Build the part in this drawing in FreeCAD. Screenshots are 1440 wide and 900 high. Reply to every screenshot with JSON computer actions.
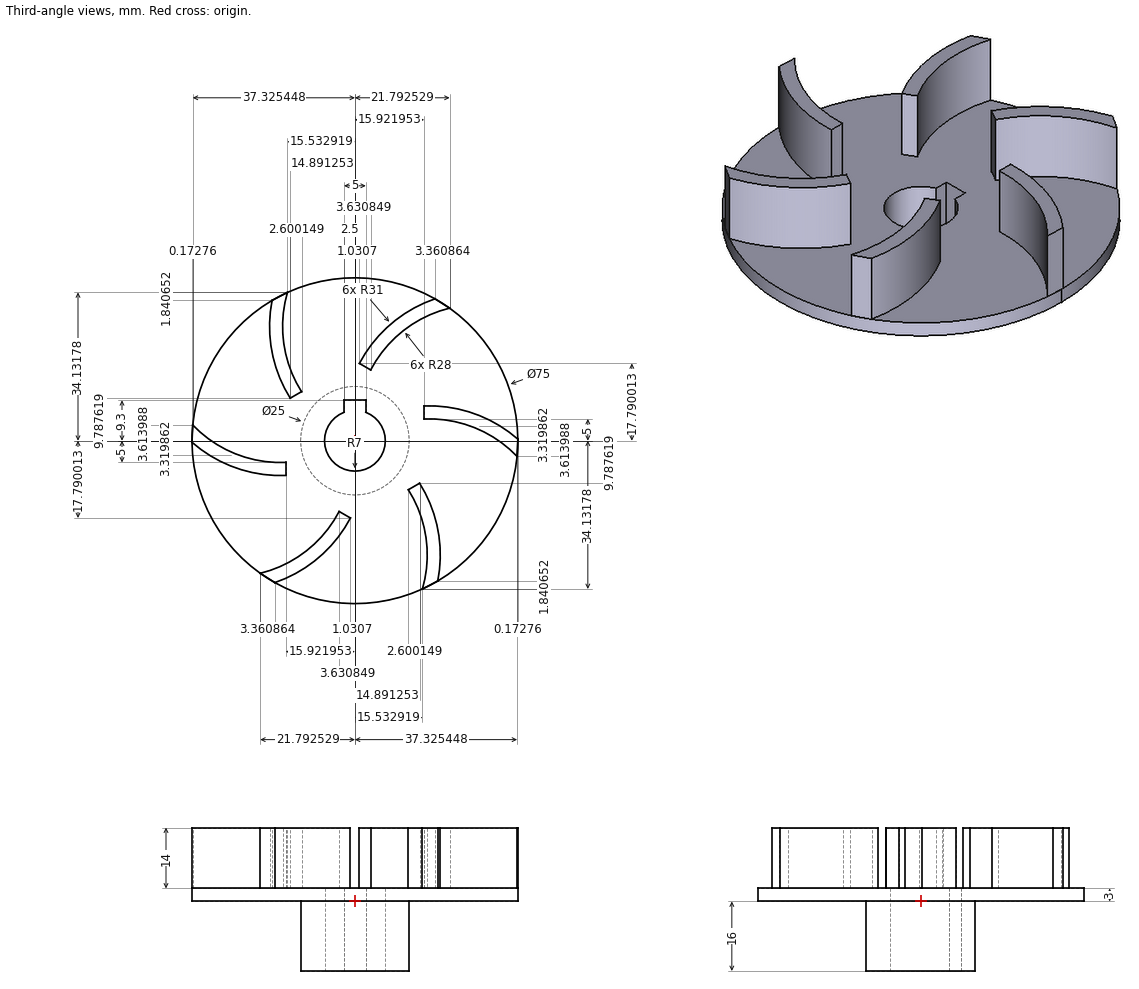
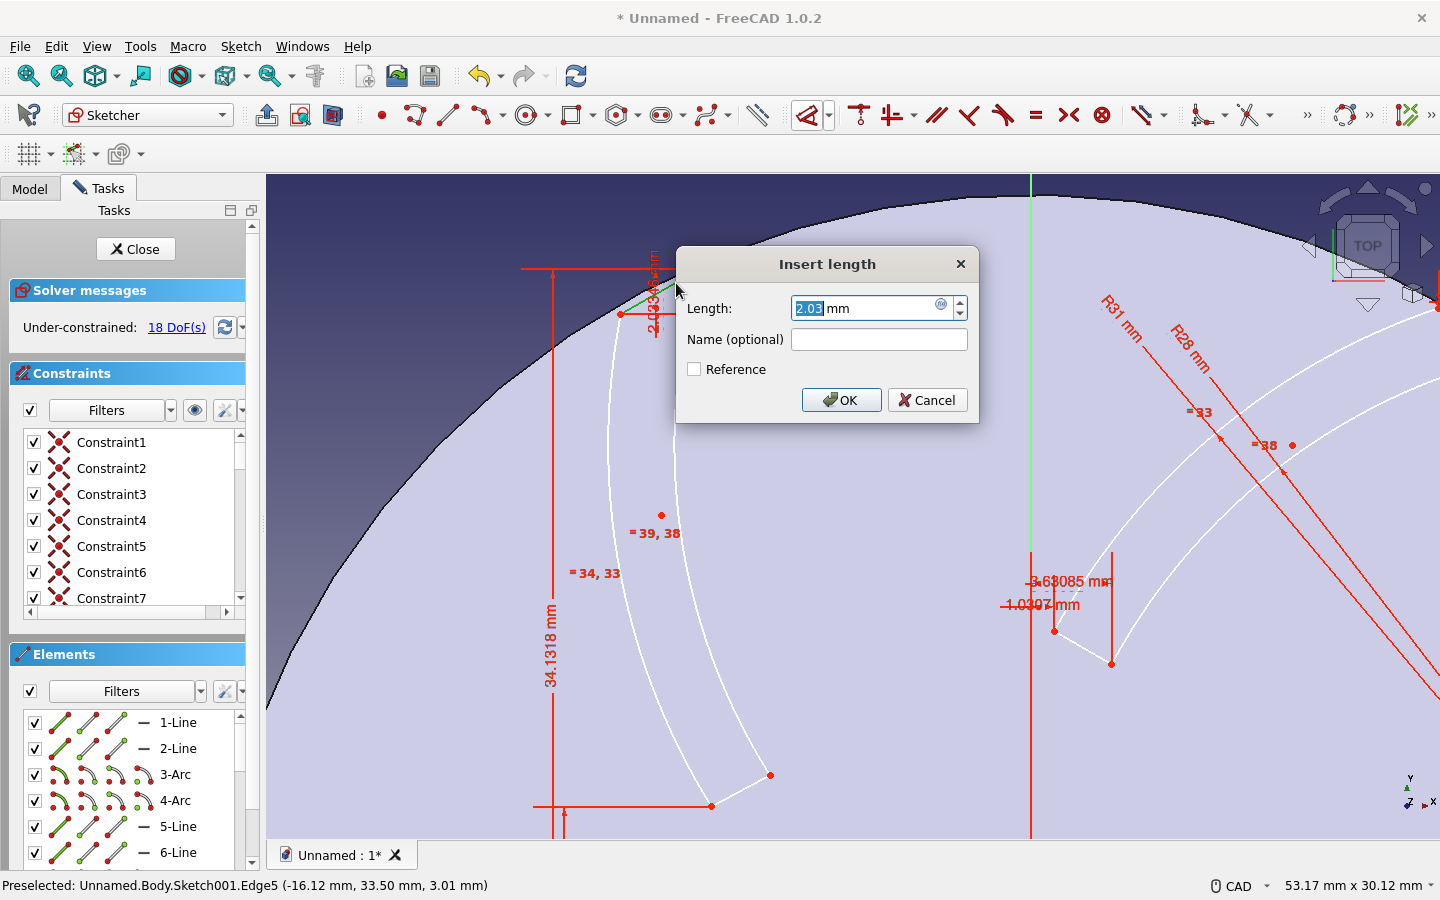
{"action": "type", "text": "1.840652"}
{"action": "key", "text": "Return"}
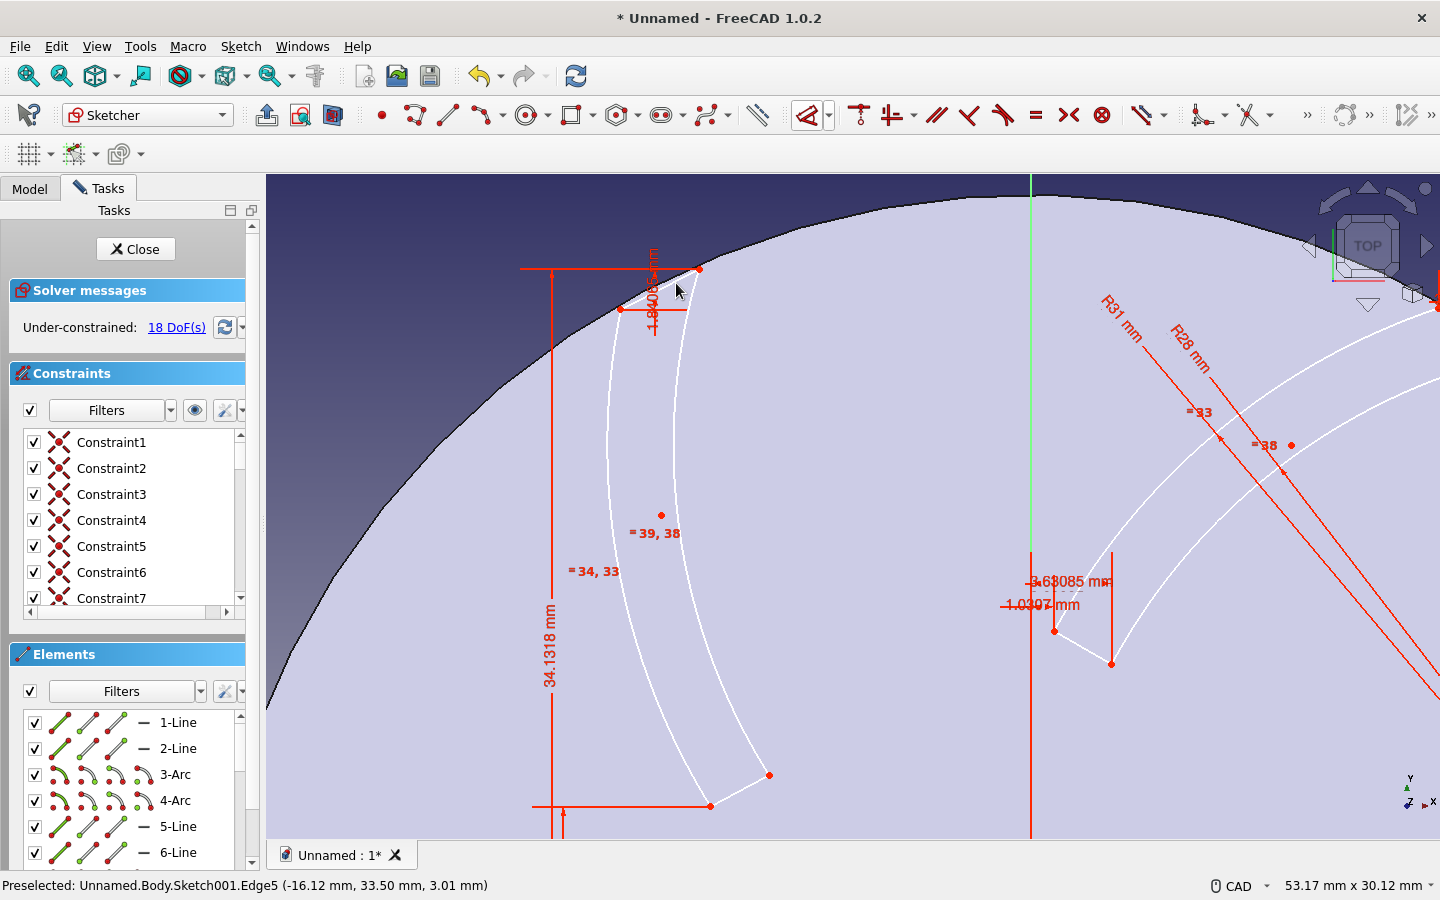
{"action": "left_click", "coordinate": [728, 797]}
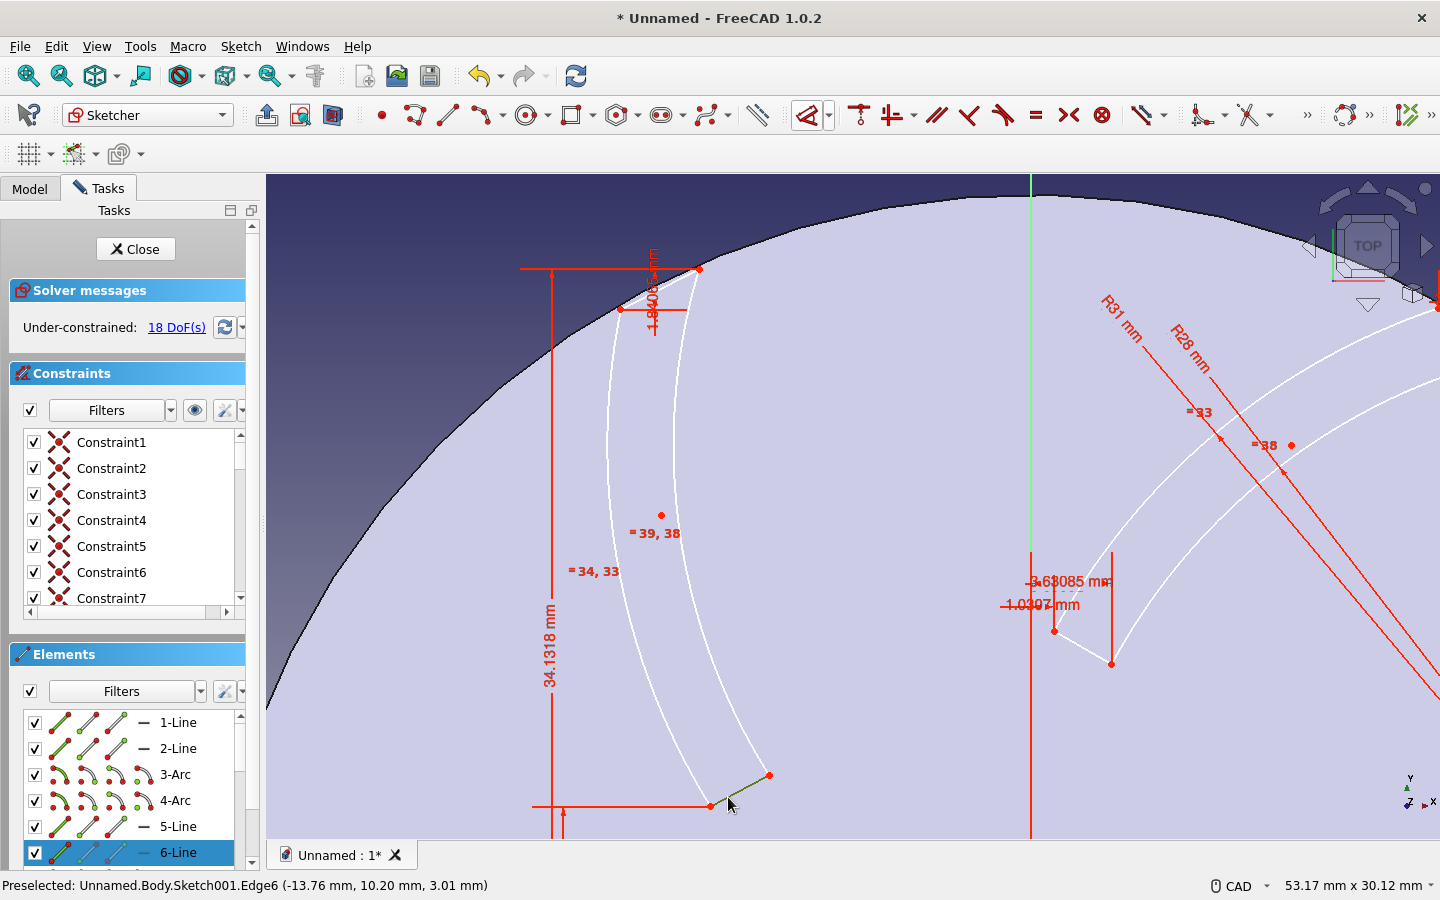
{"action": "key", "text": "l"}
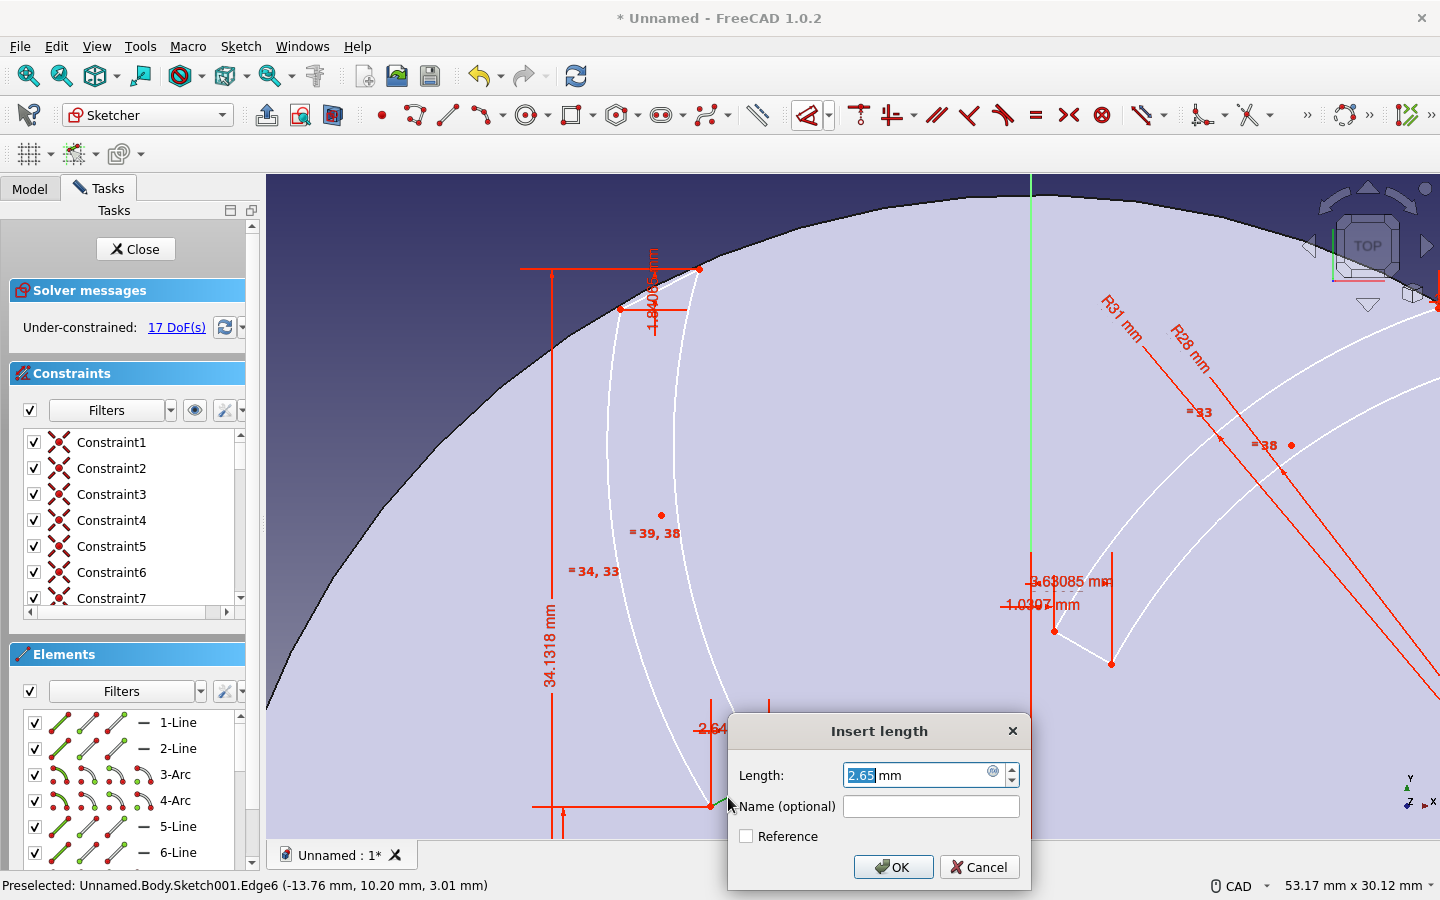
{"action": "type", "text": "2.600149"}
{"action": "key", "text": "Return"}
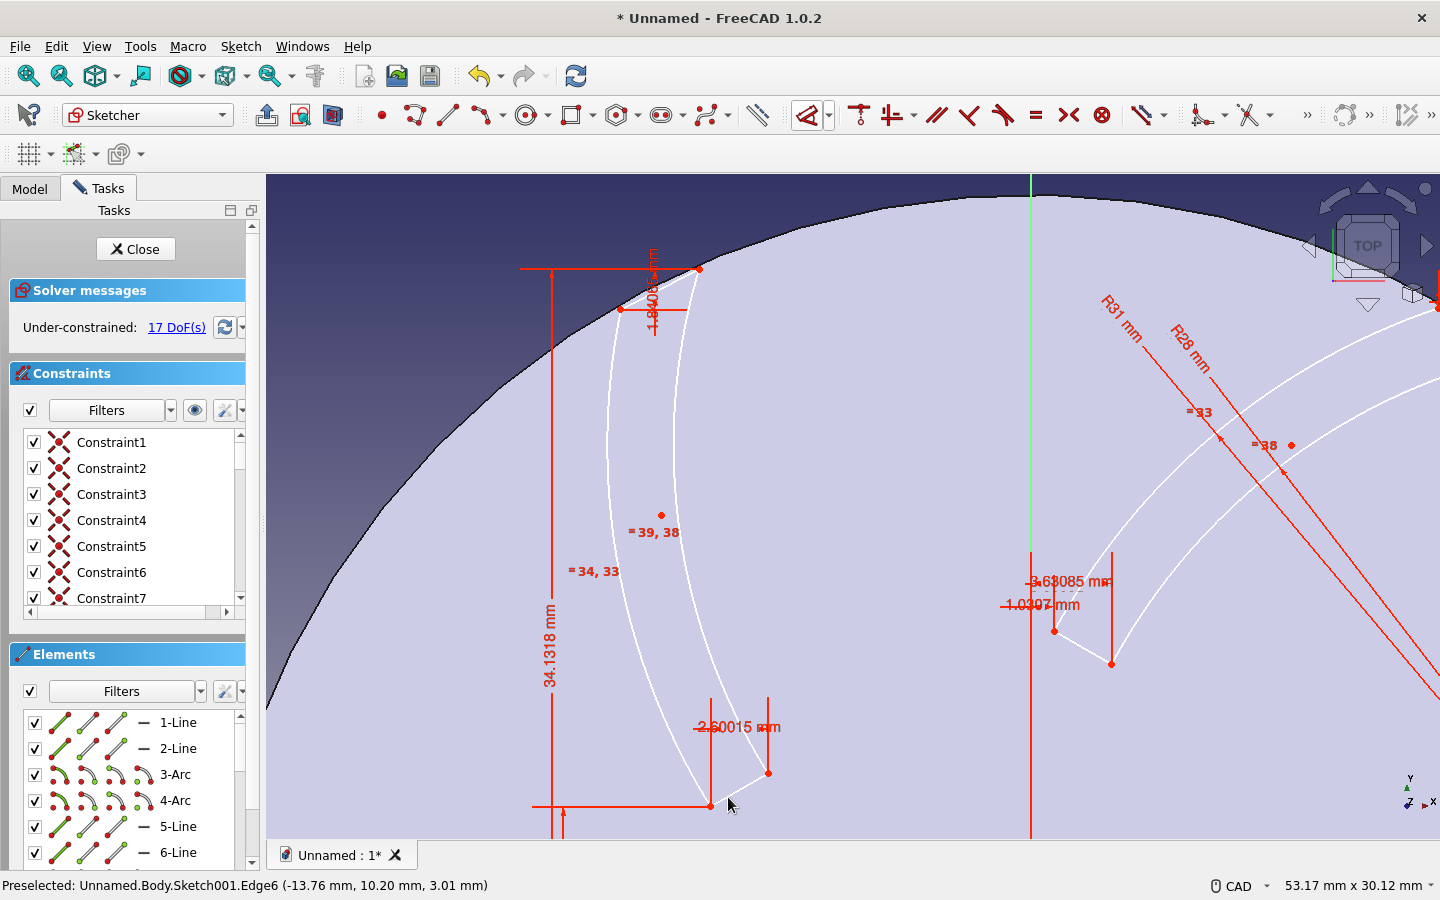
{"action": "scroll", "coordinate": [678, 284], "scroll_direction": "down", "scroll_amount": 6}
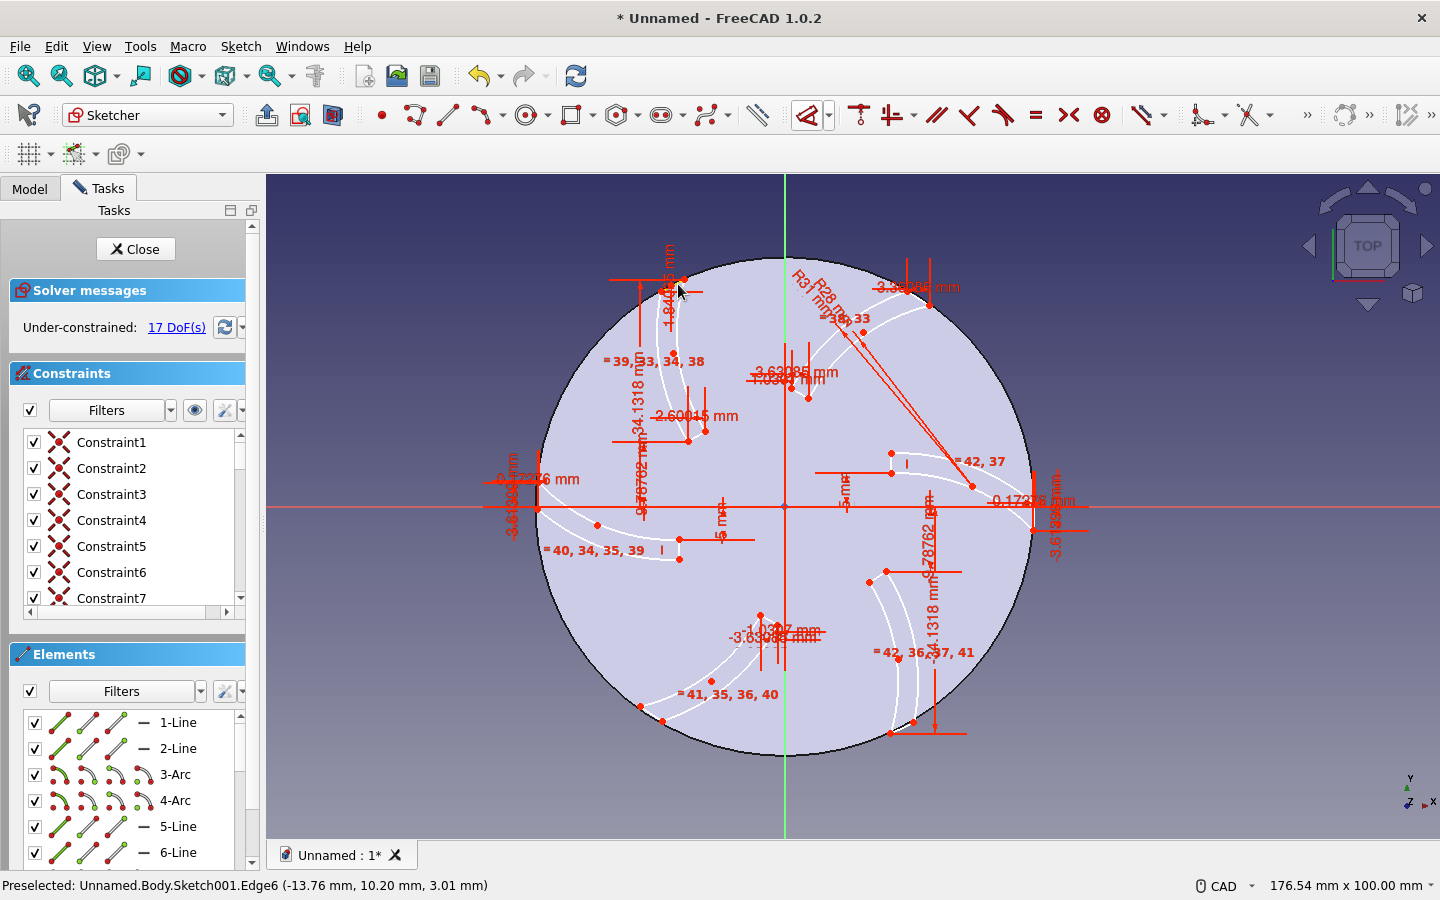
{"action": "scroll", "coordinate": [647, 711], "scroll_direction": "up", "scroll_amount": 5}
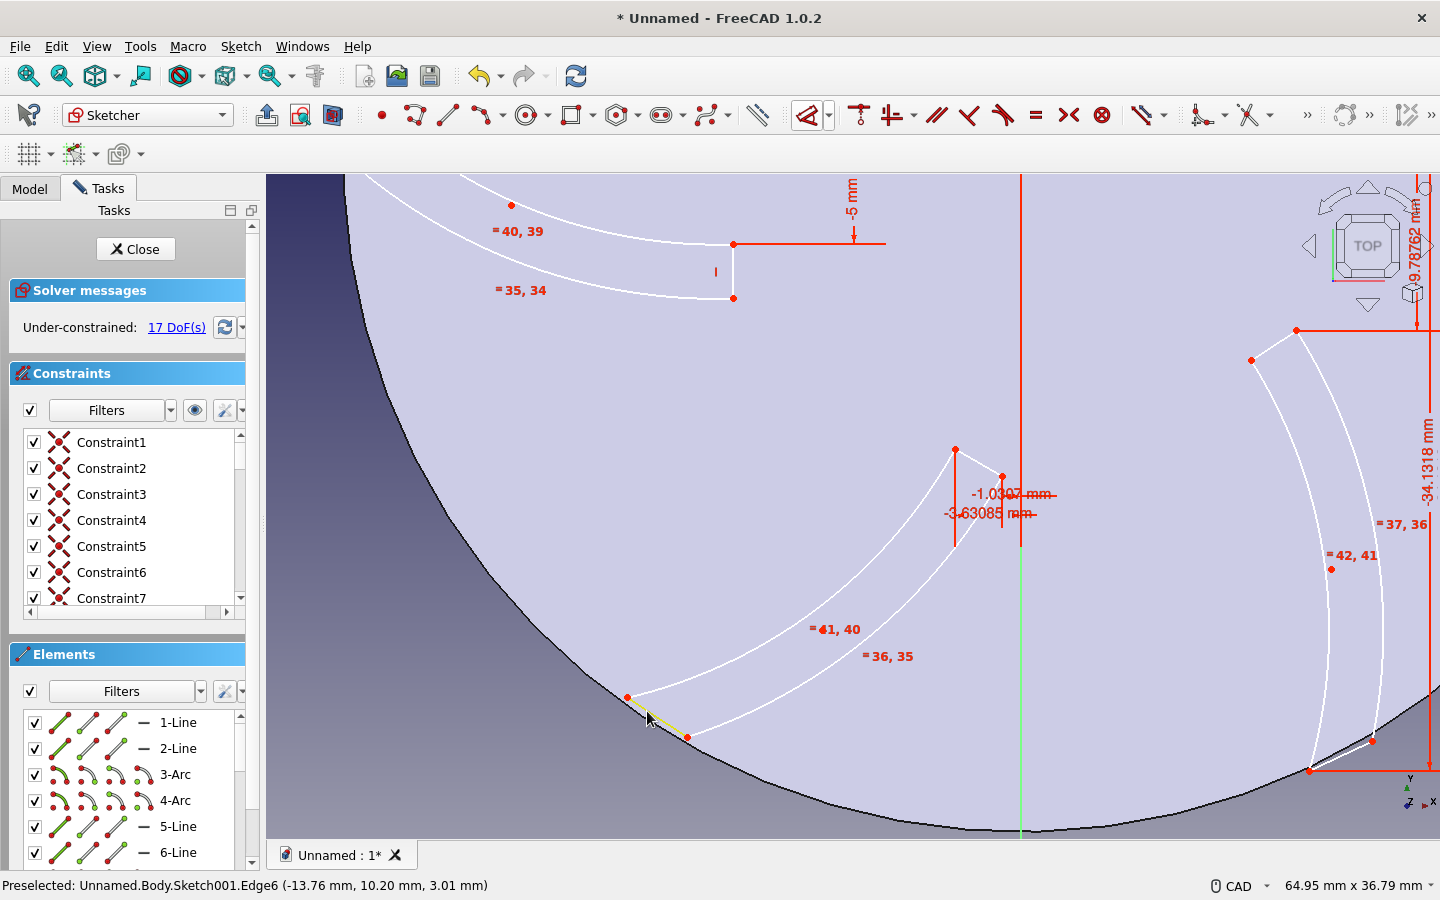
{"action": "left_click", "coordinate": [645, 710]}